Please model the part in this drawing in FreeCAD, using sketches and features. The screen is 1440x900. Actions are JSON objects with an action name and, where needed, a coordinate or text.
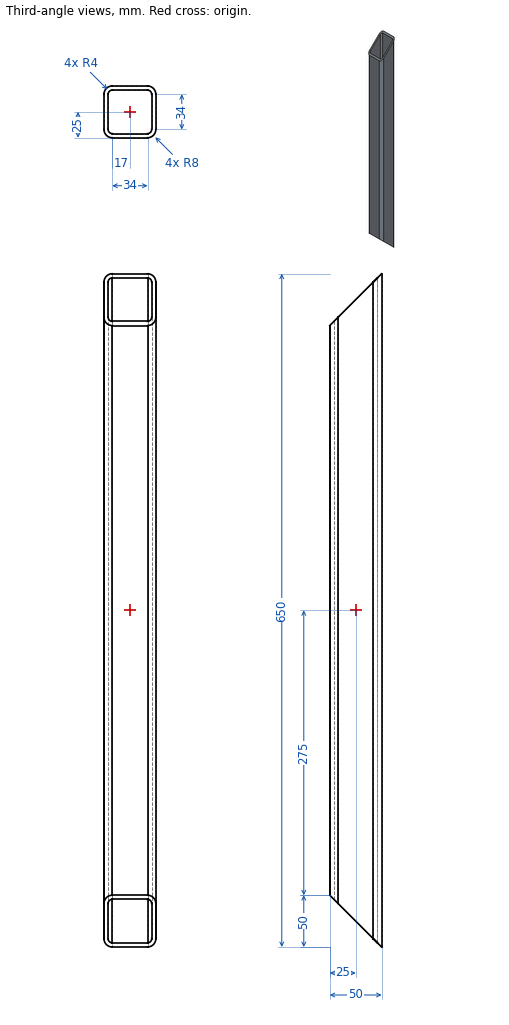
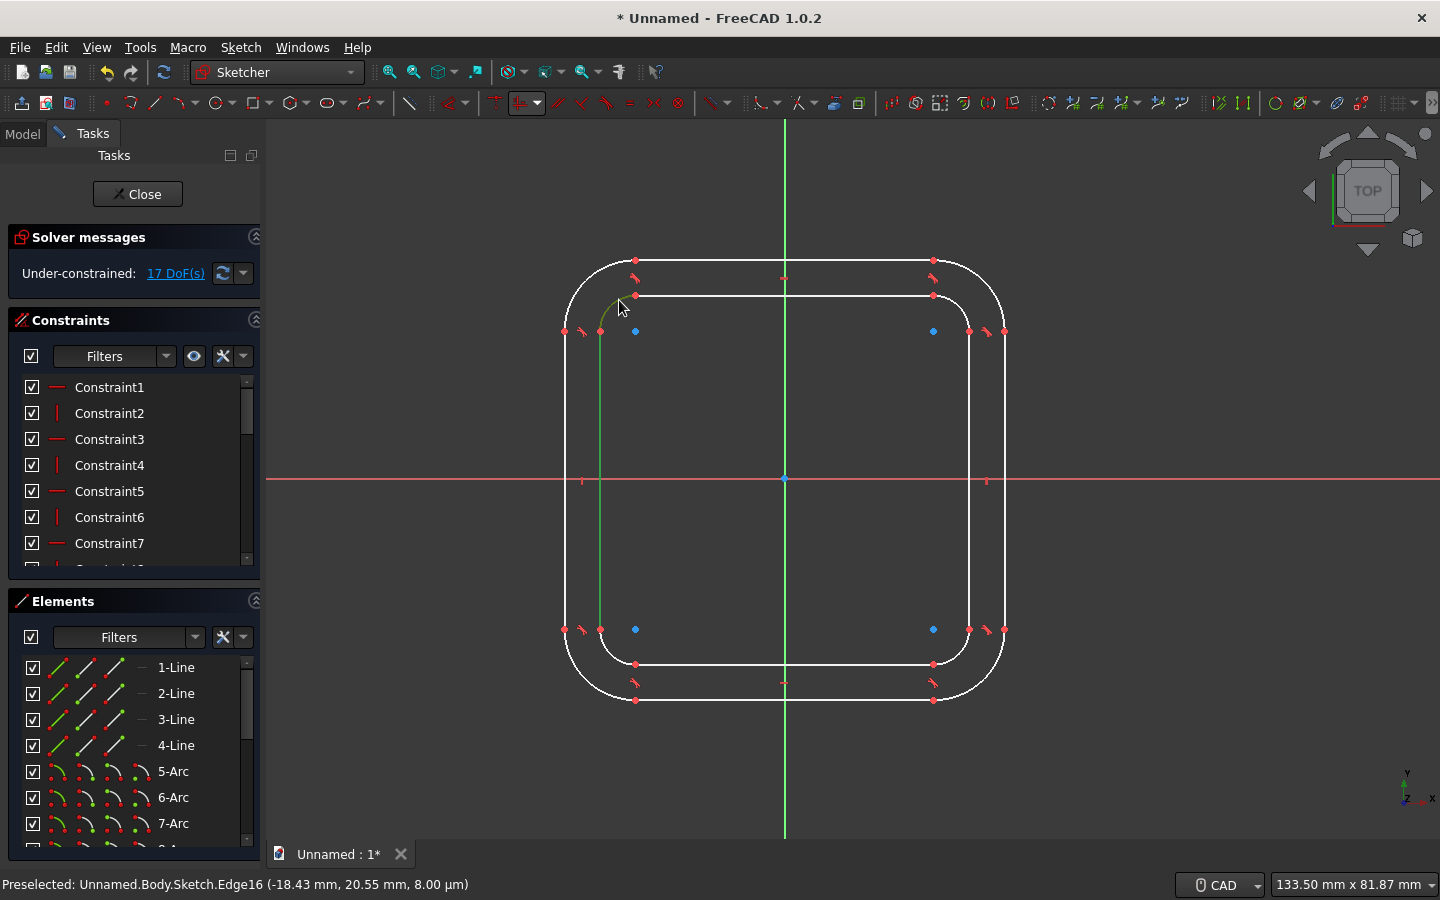
{"action": "left_click", "coordinate": [606, 104]}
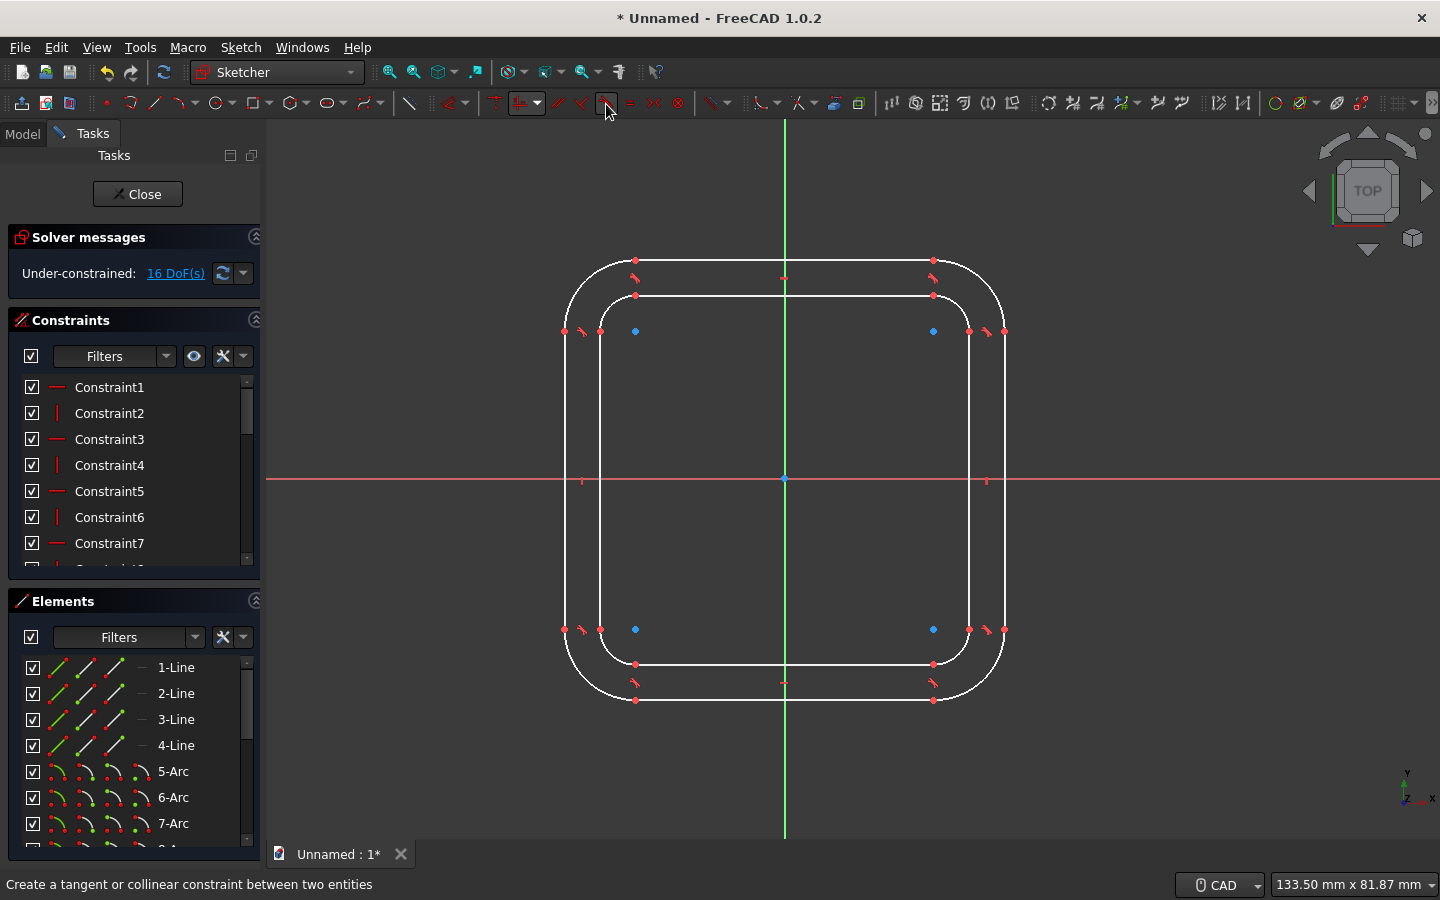
{"action": "left_click", "coordinate": [997, 299]}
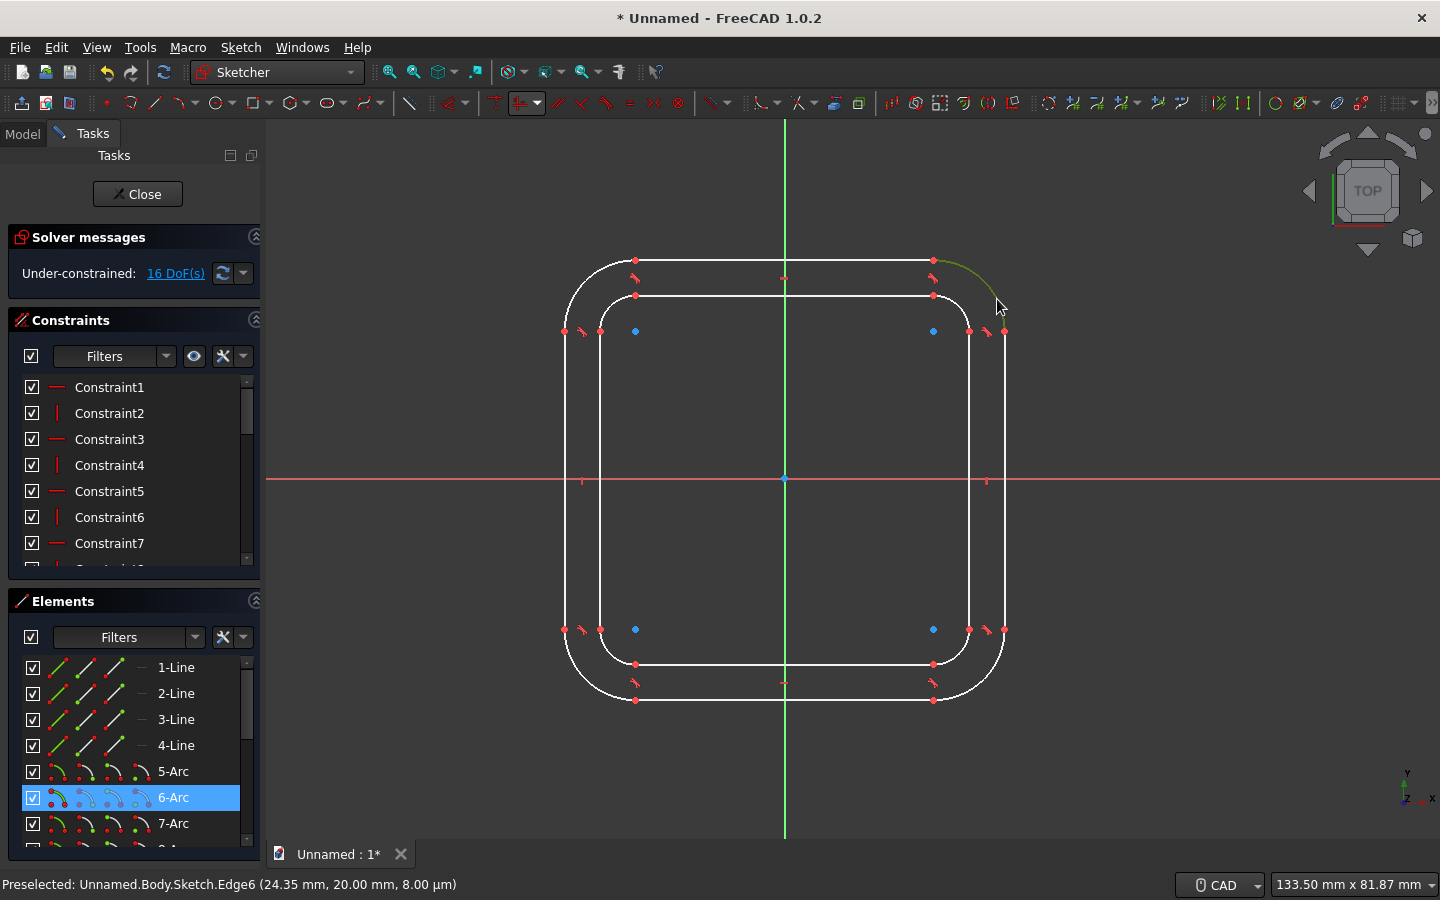
{"action": "left_click", "coordinate": [965, 315]}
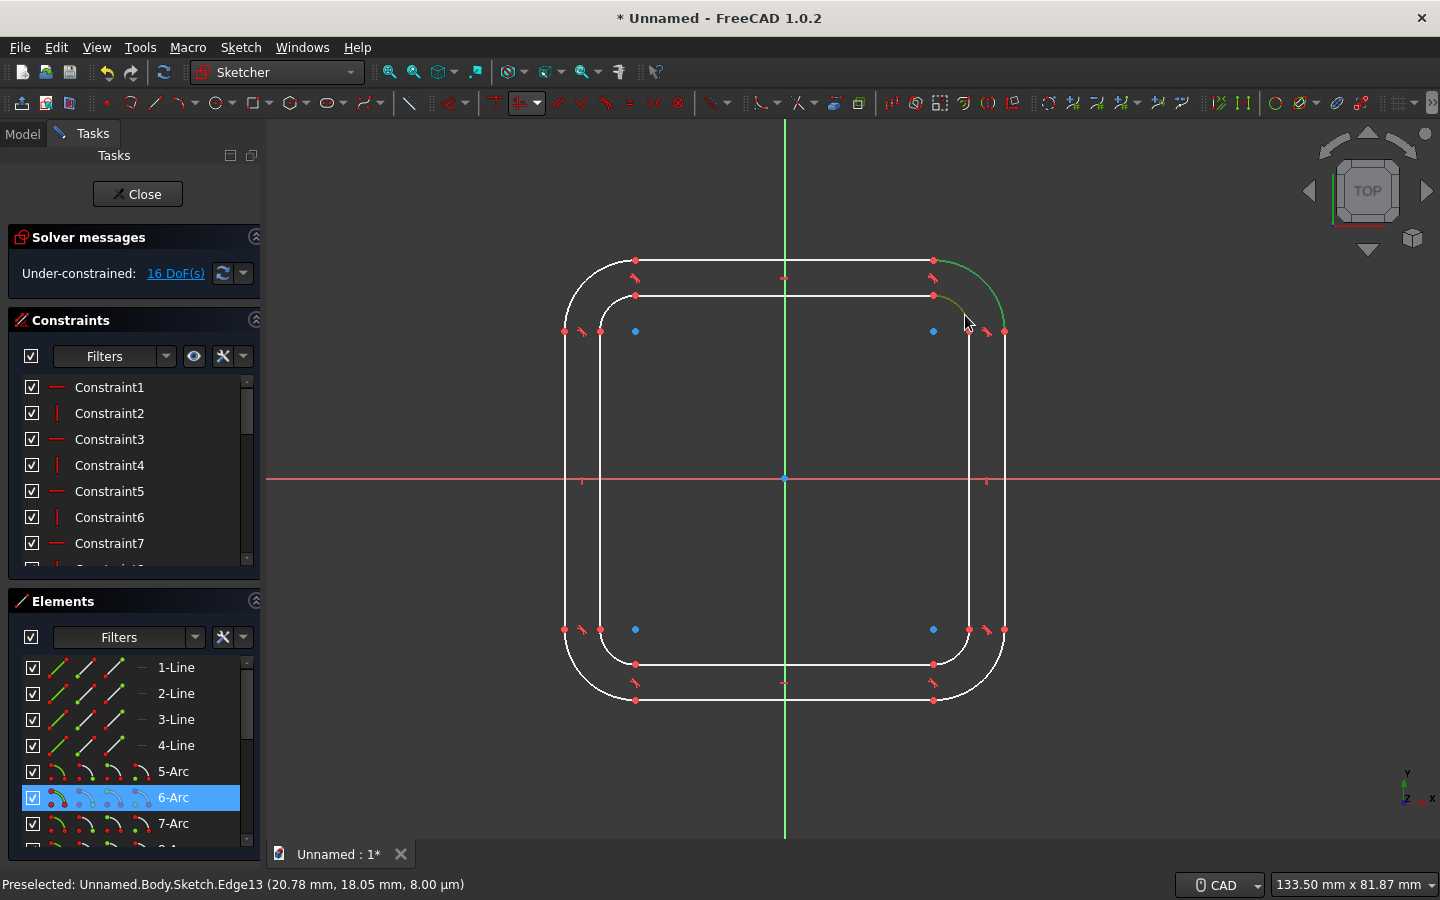
{"action": "left_click", "coordinate": [496, 104]}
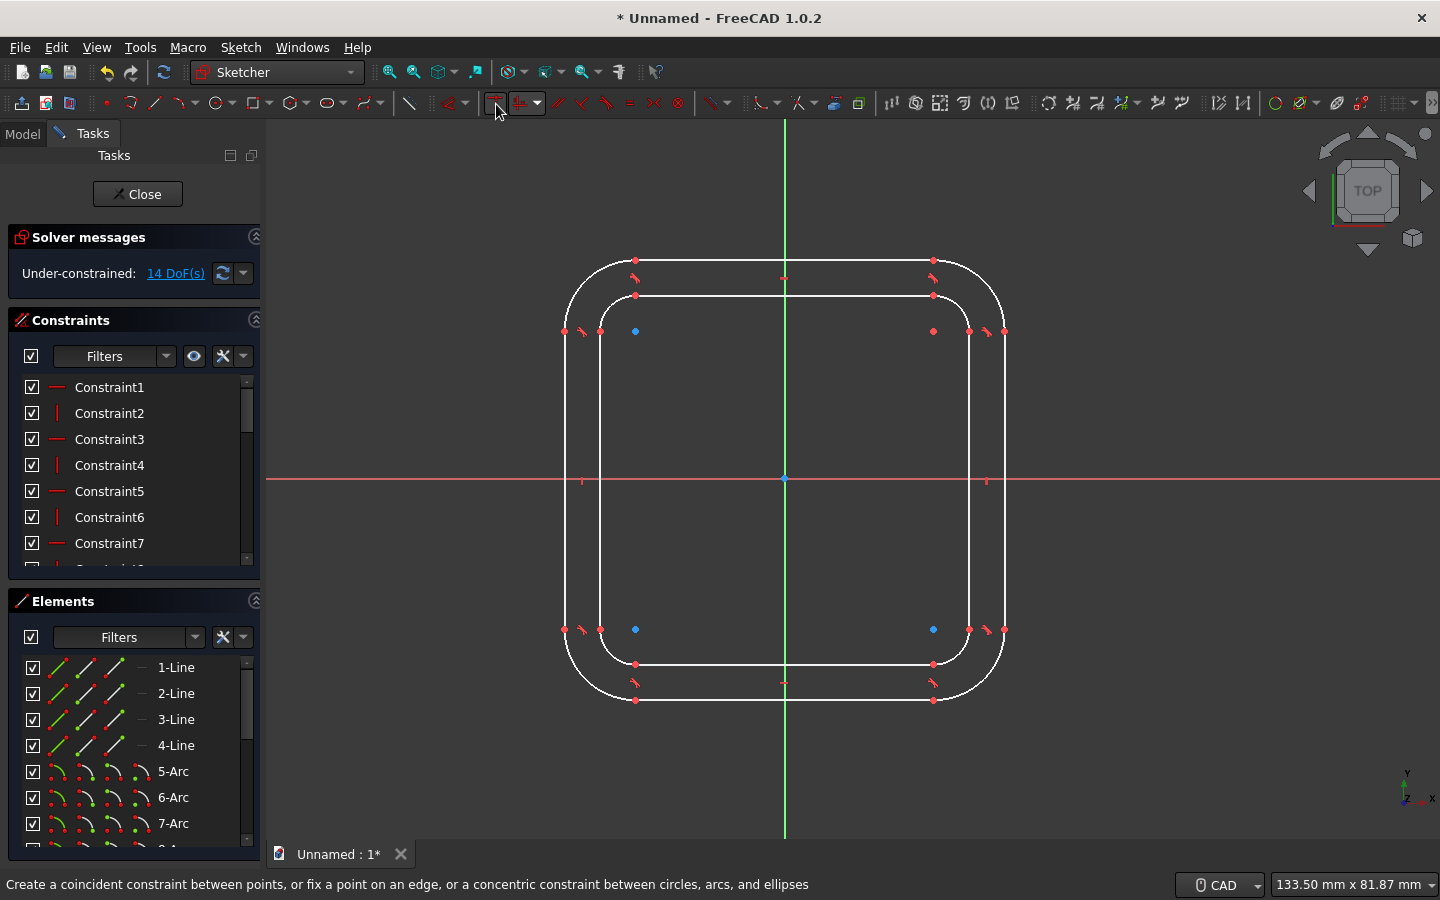
{"action": "left_click", "coordinate": [966, 692]}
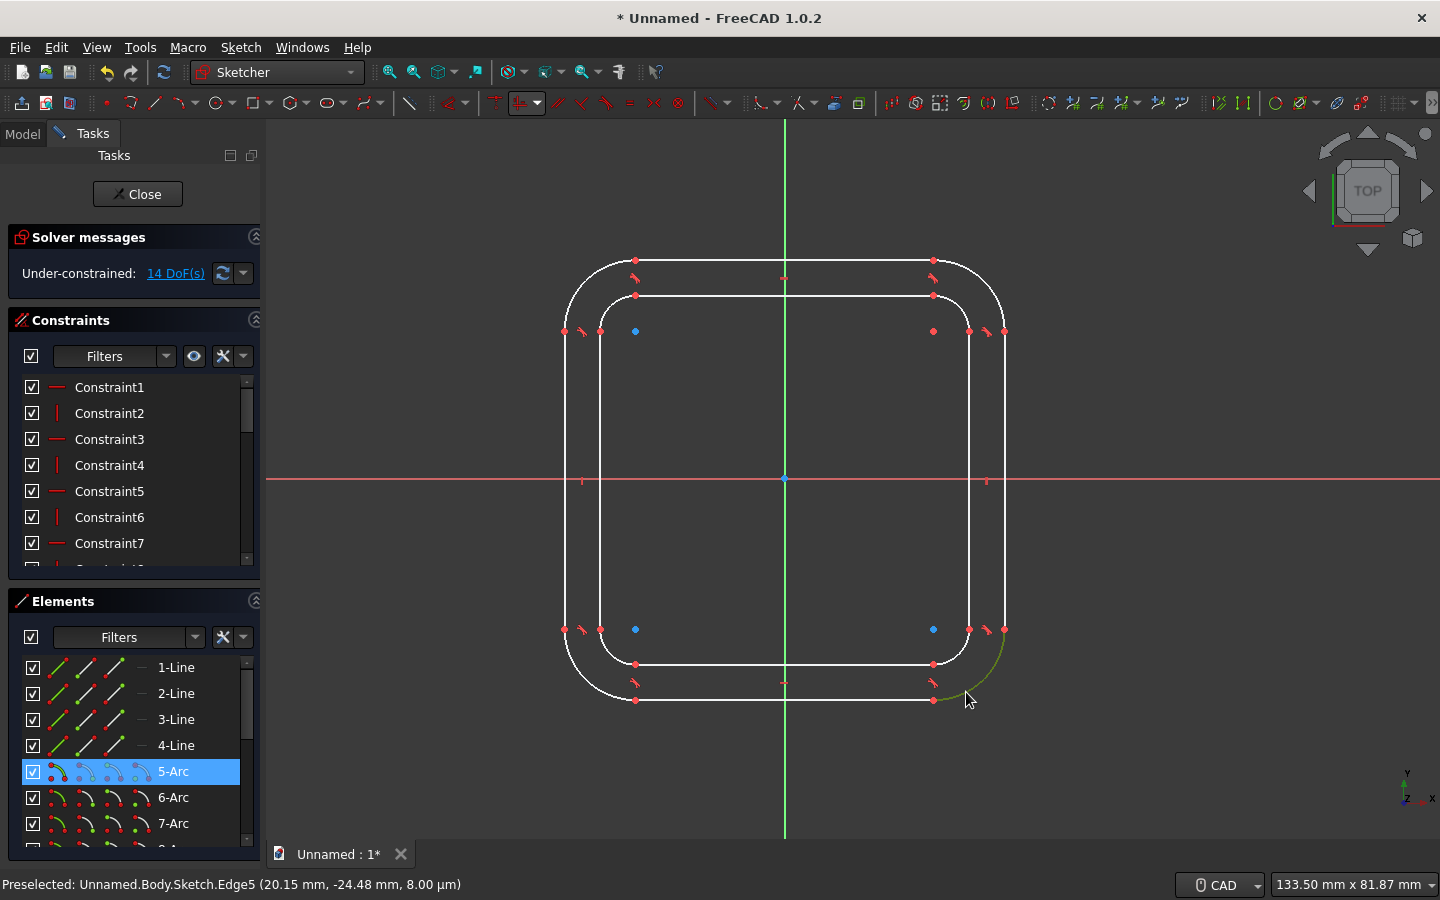
{"action": "left_click", "coordinate": [950, 661]}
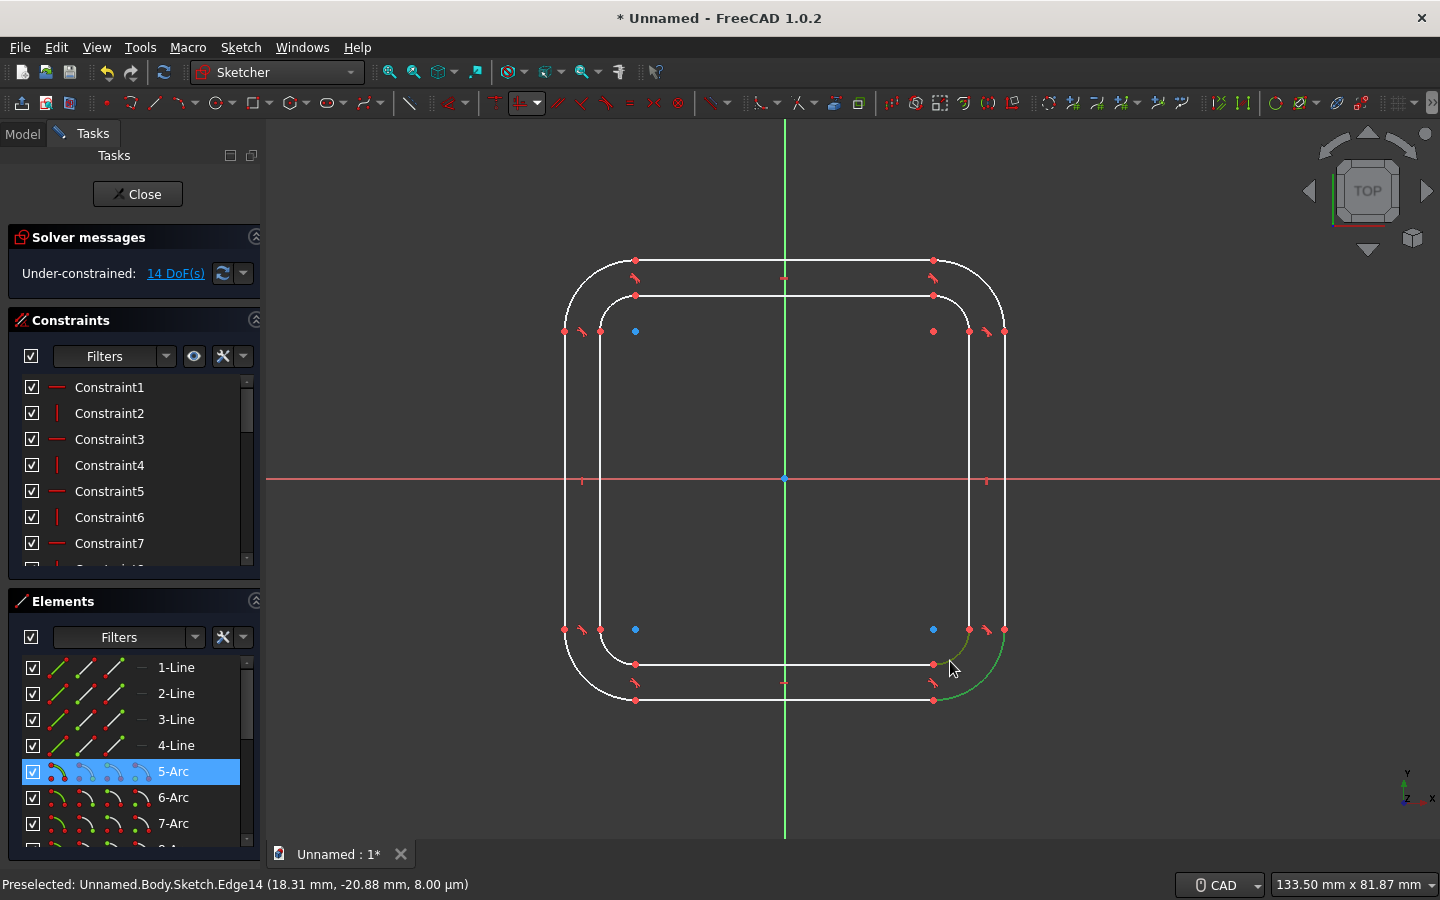
{"action": "left_click", "coordinate": [496, 104]}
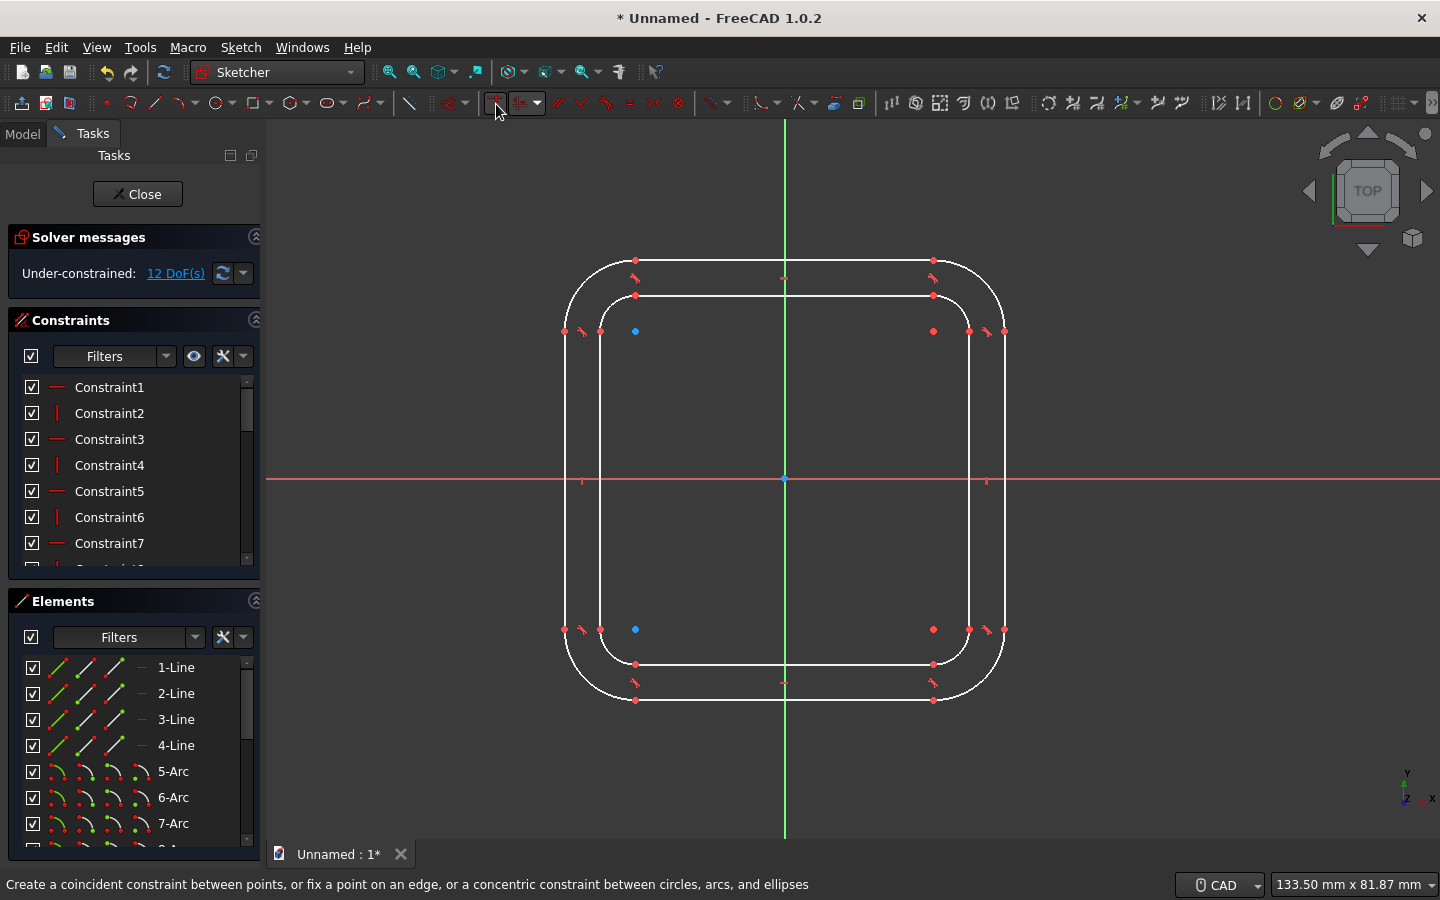
{"action": "left_click", "coordinate": [573, 661]}